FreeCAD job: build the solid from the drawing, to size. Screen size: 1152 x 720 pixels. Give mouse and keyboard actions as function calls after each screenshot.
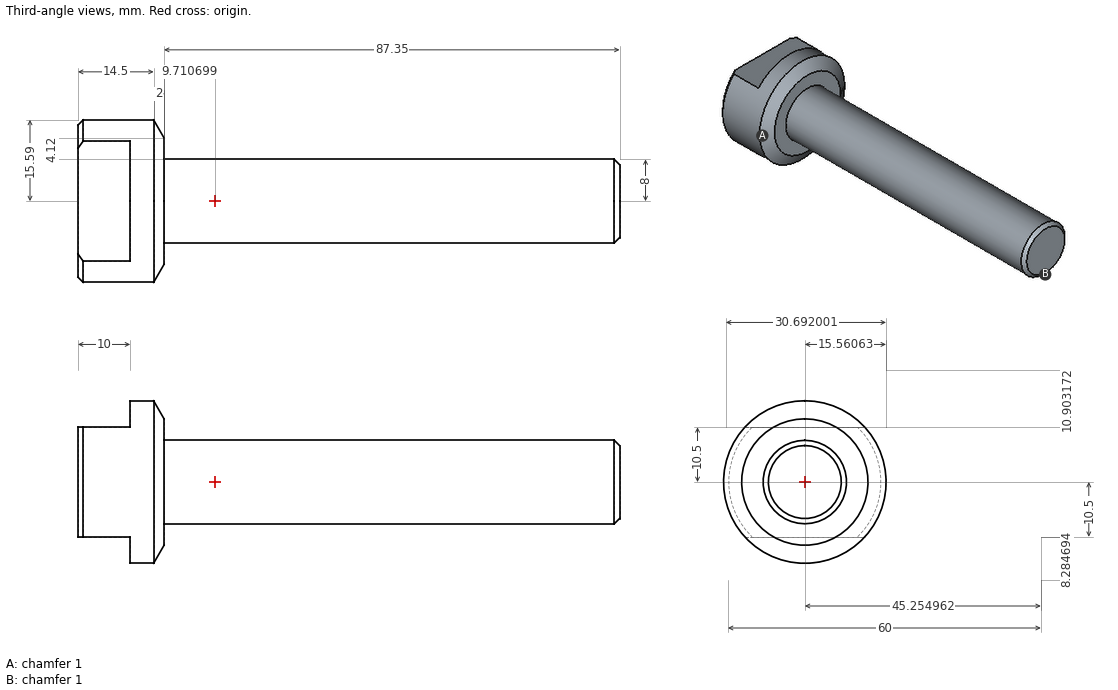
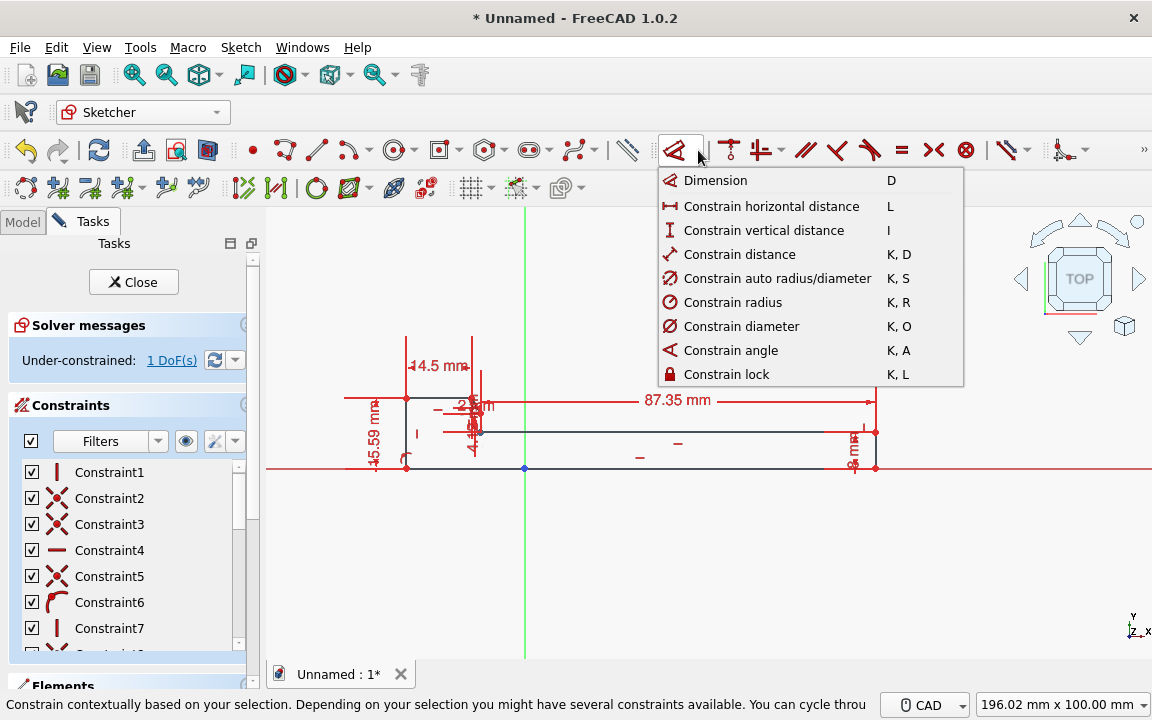
click(811, 206)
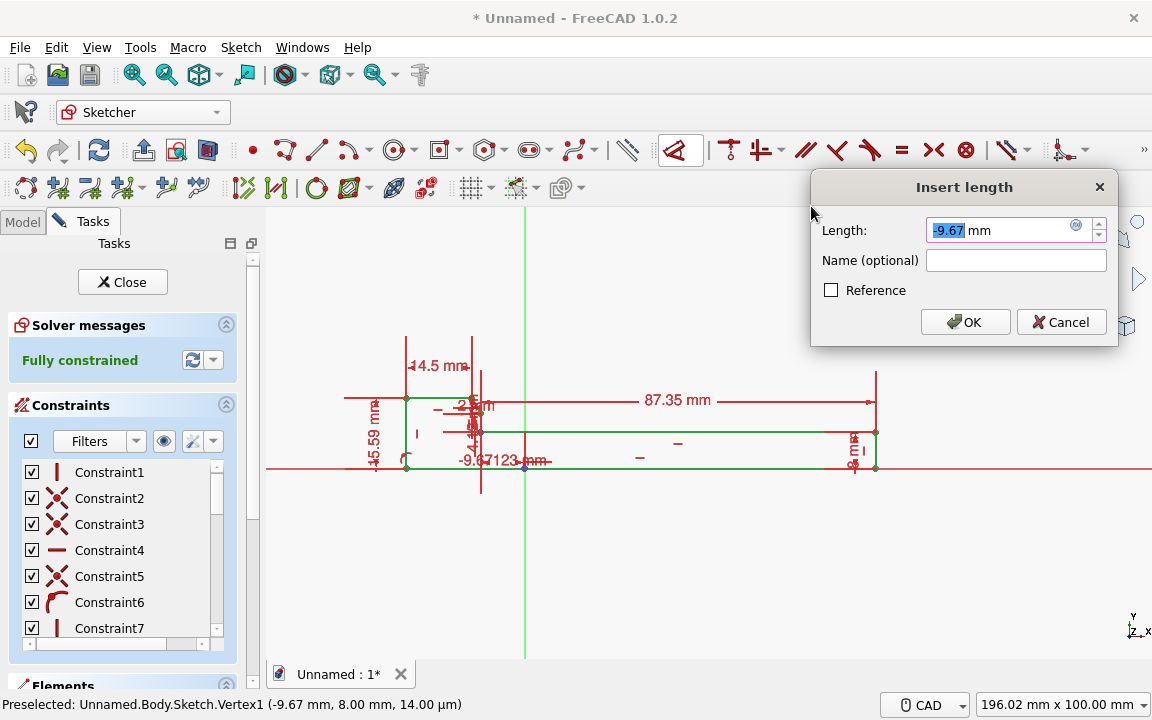
text(-9.710699)
key(Return)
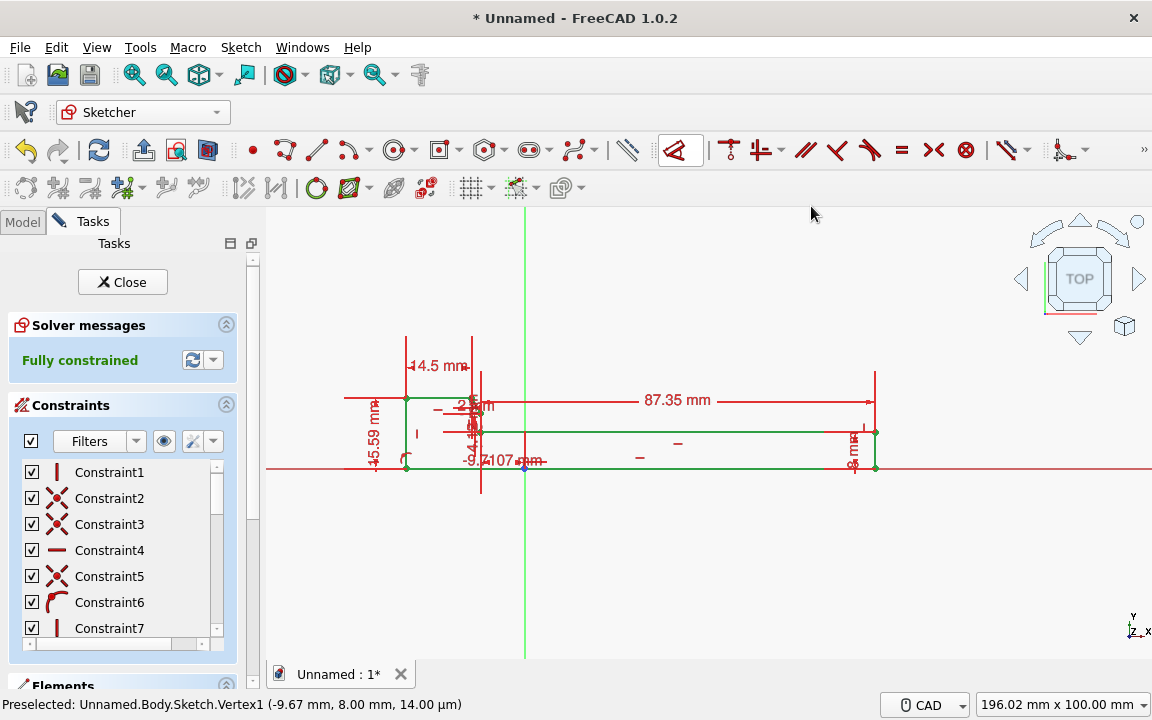
click(123, 282)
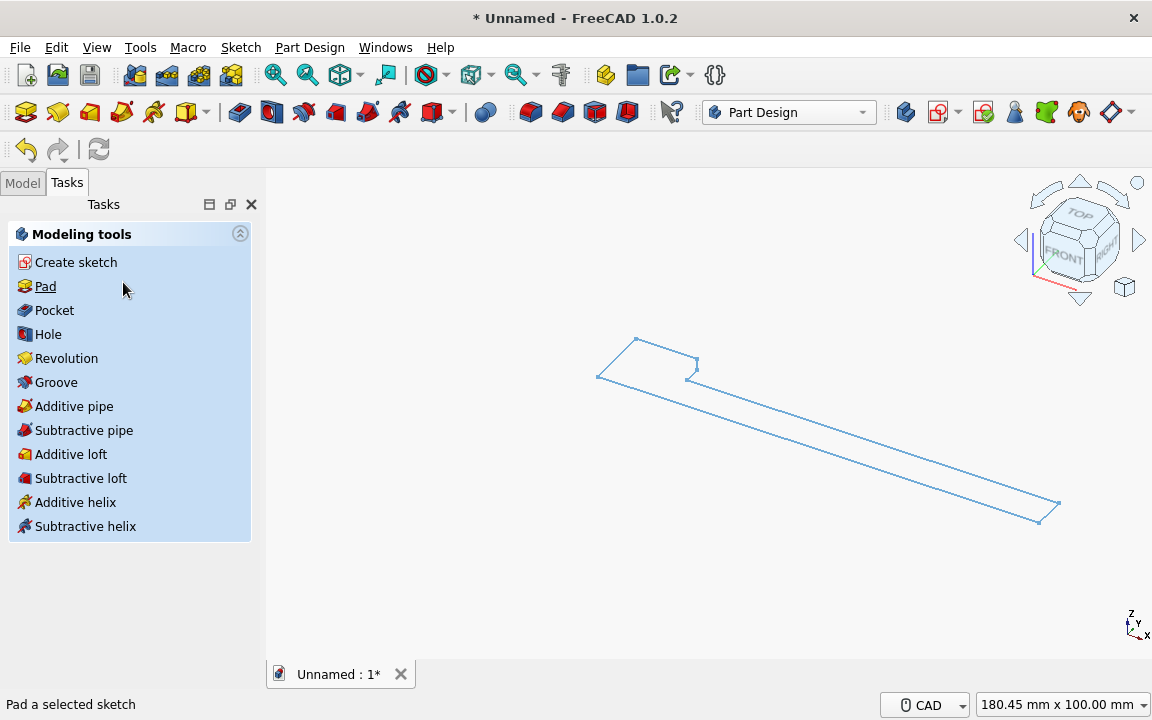
click(58, 112)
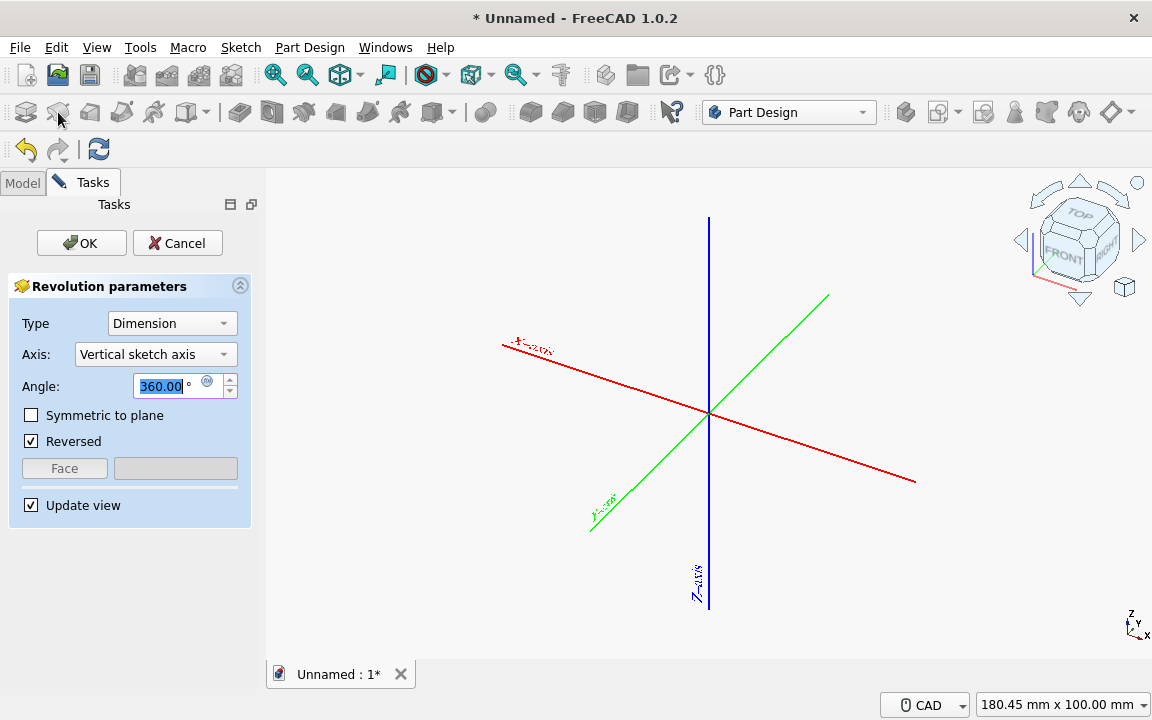
click(156, 354)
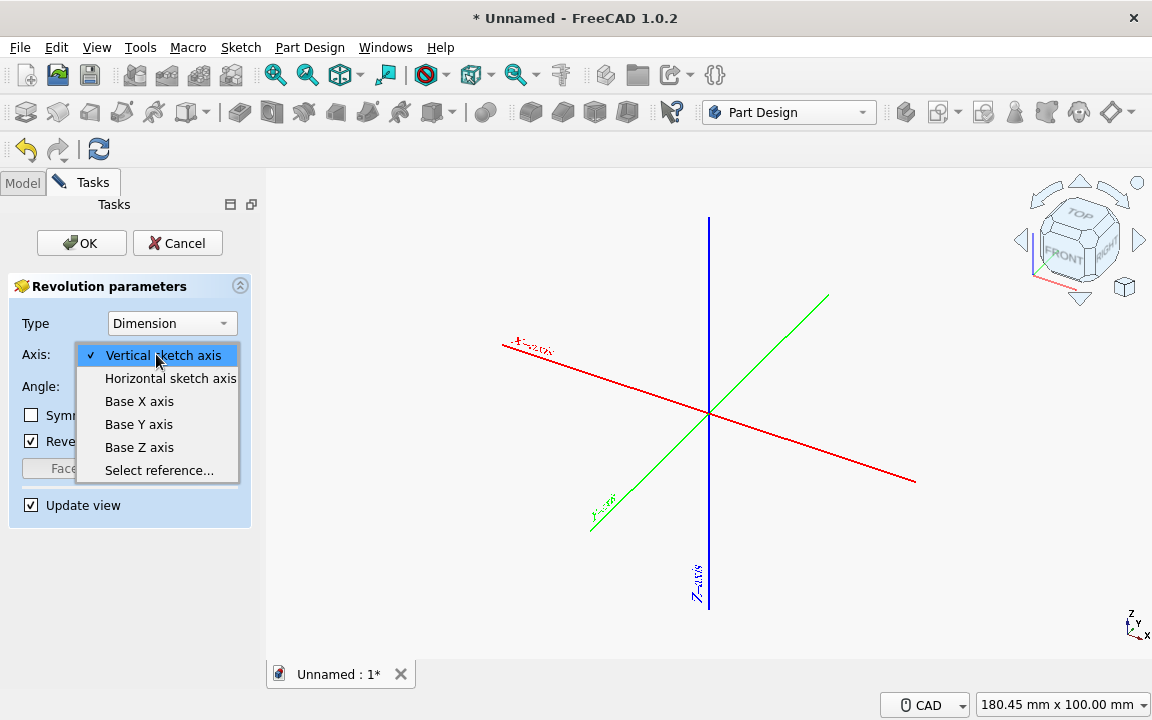
click(156, 378)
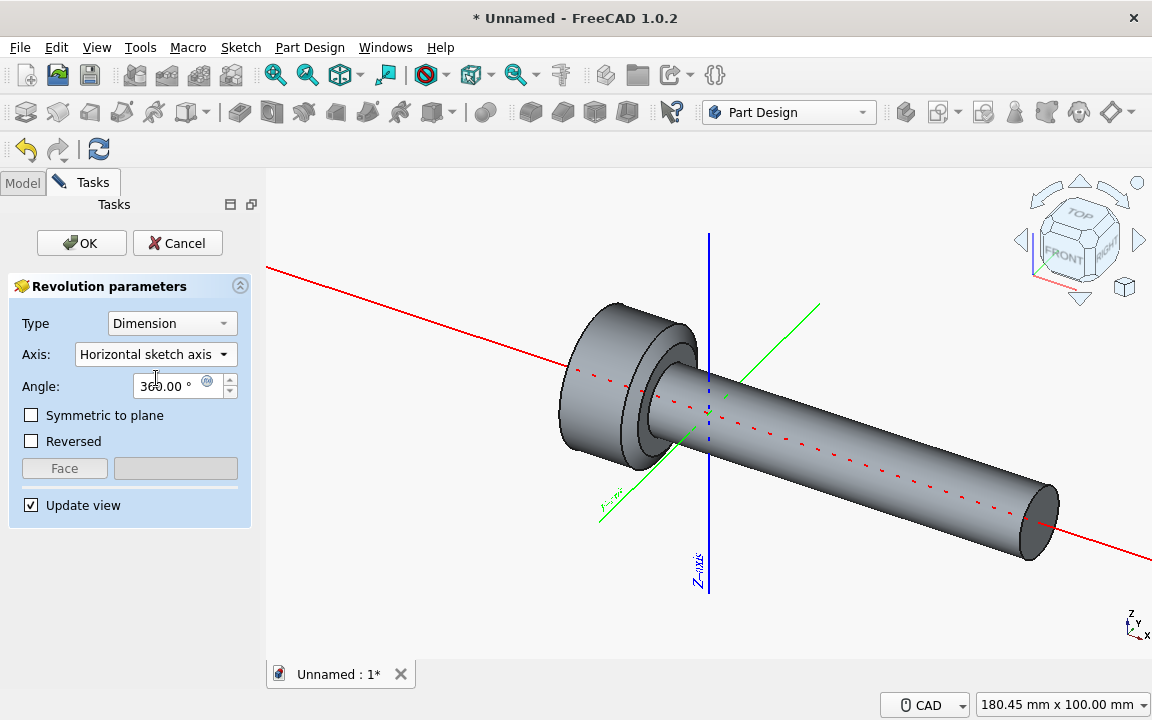
click(82, 243)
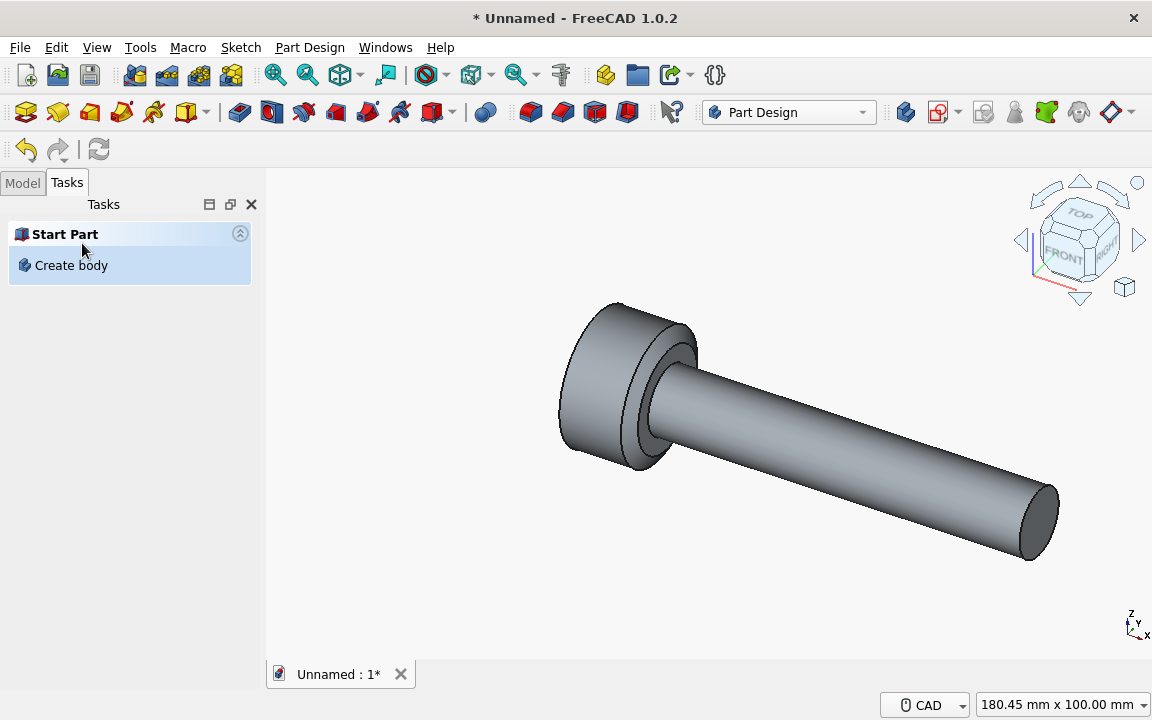
click(609, 304)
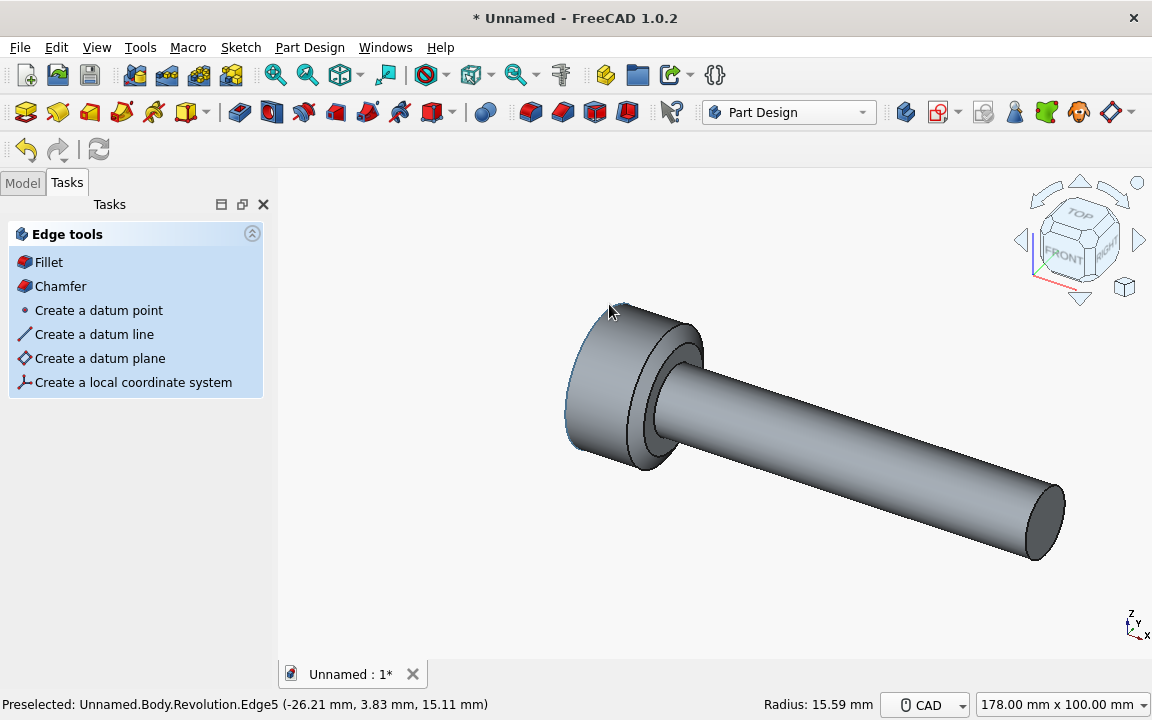
click(564, 112)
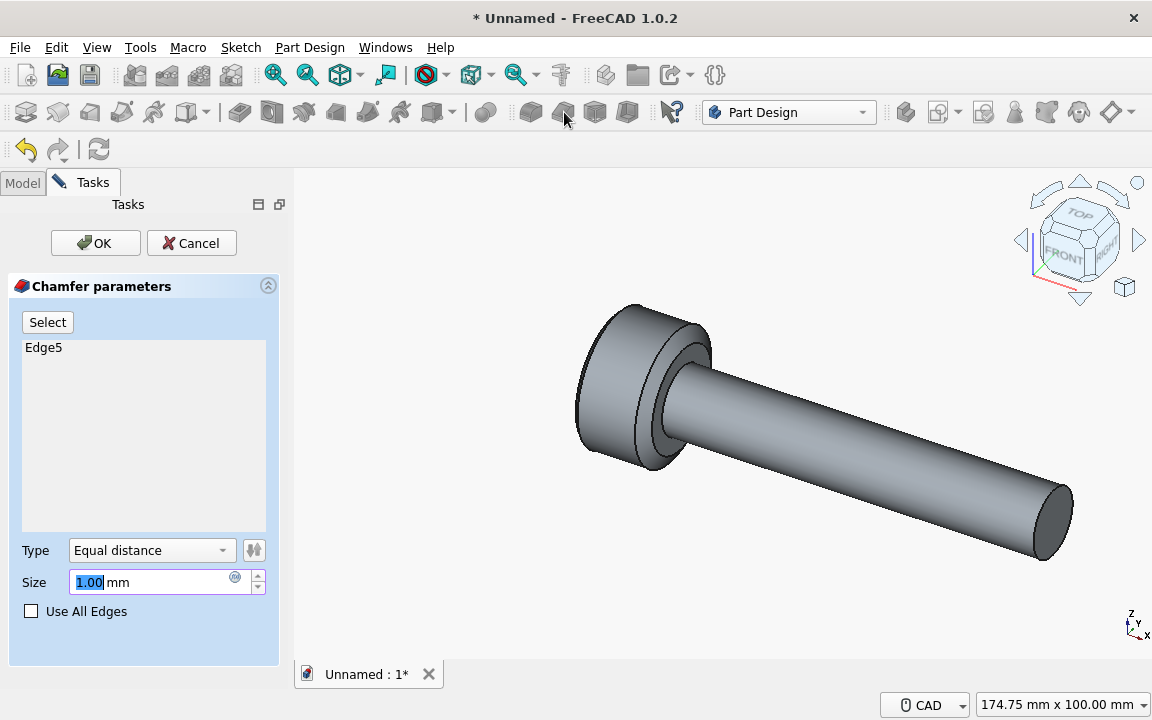
text(1)
key(Tab)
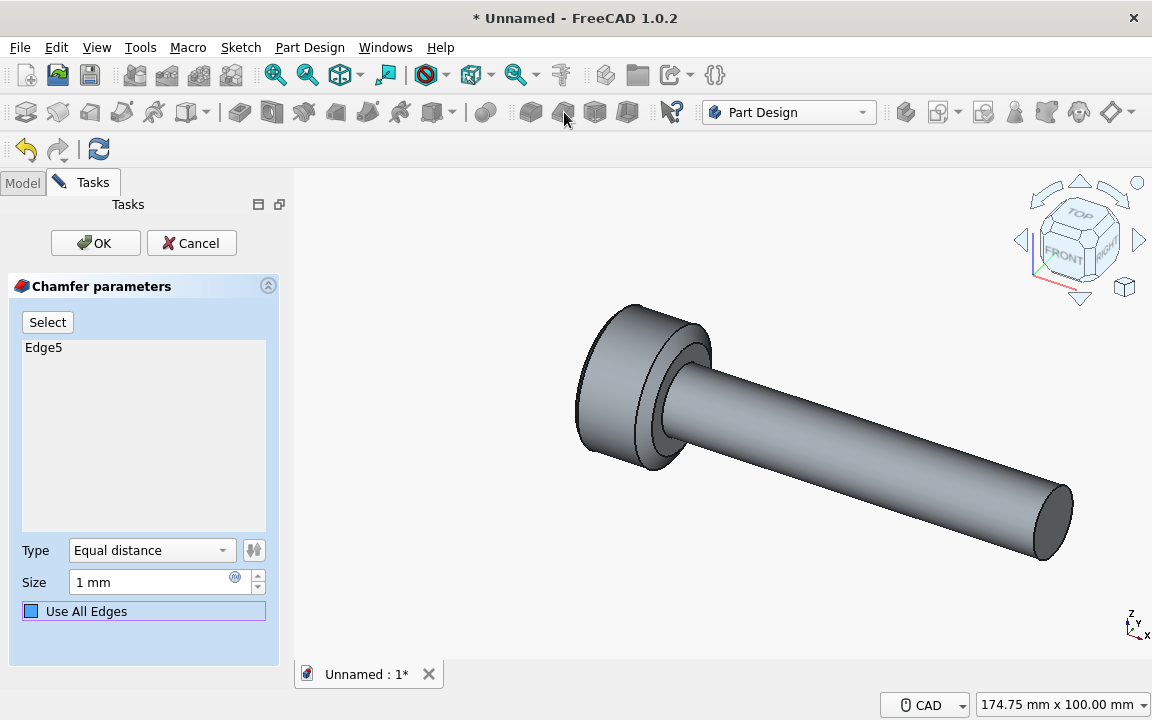
click(96, 243)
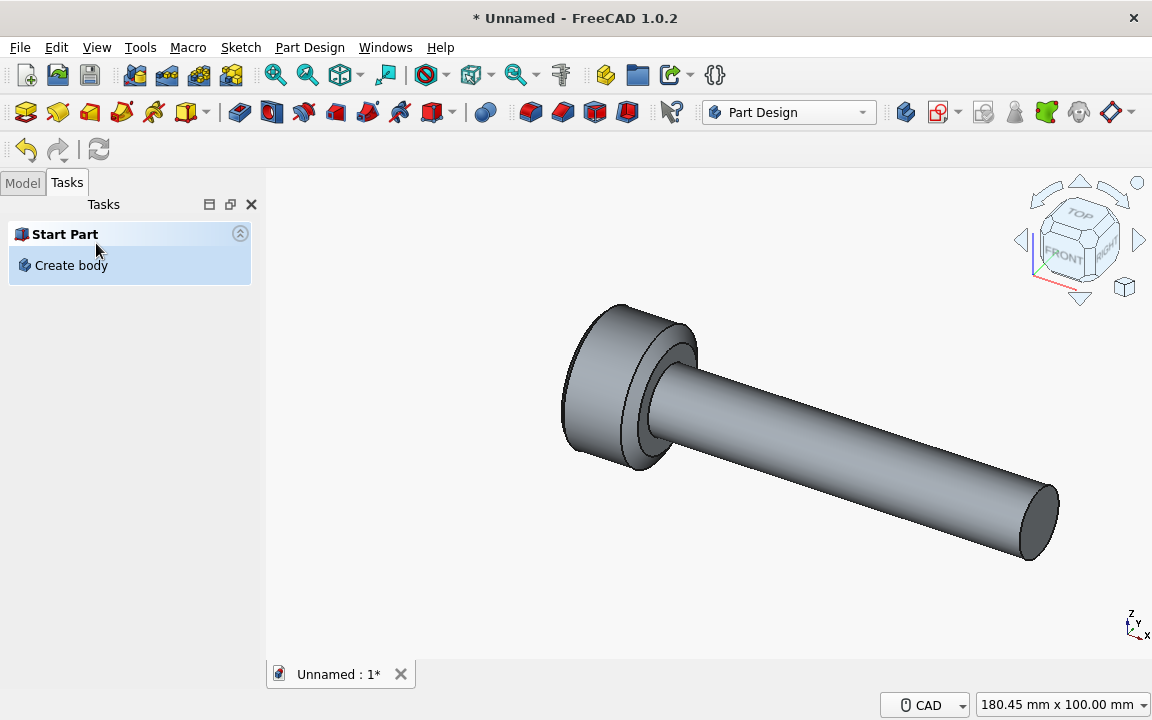
click(1019, 541)